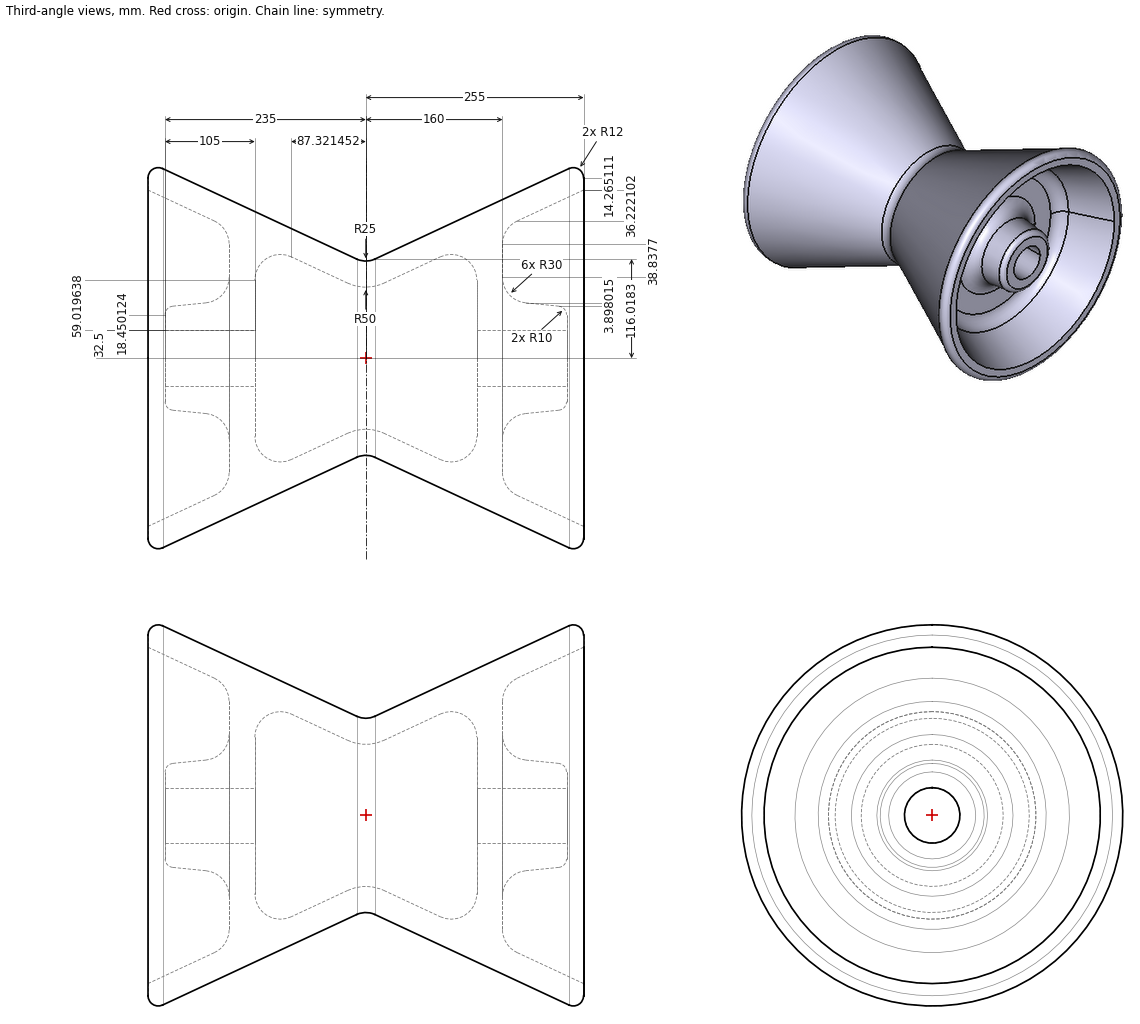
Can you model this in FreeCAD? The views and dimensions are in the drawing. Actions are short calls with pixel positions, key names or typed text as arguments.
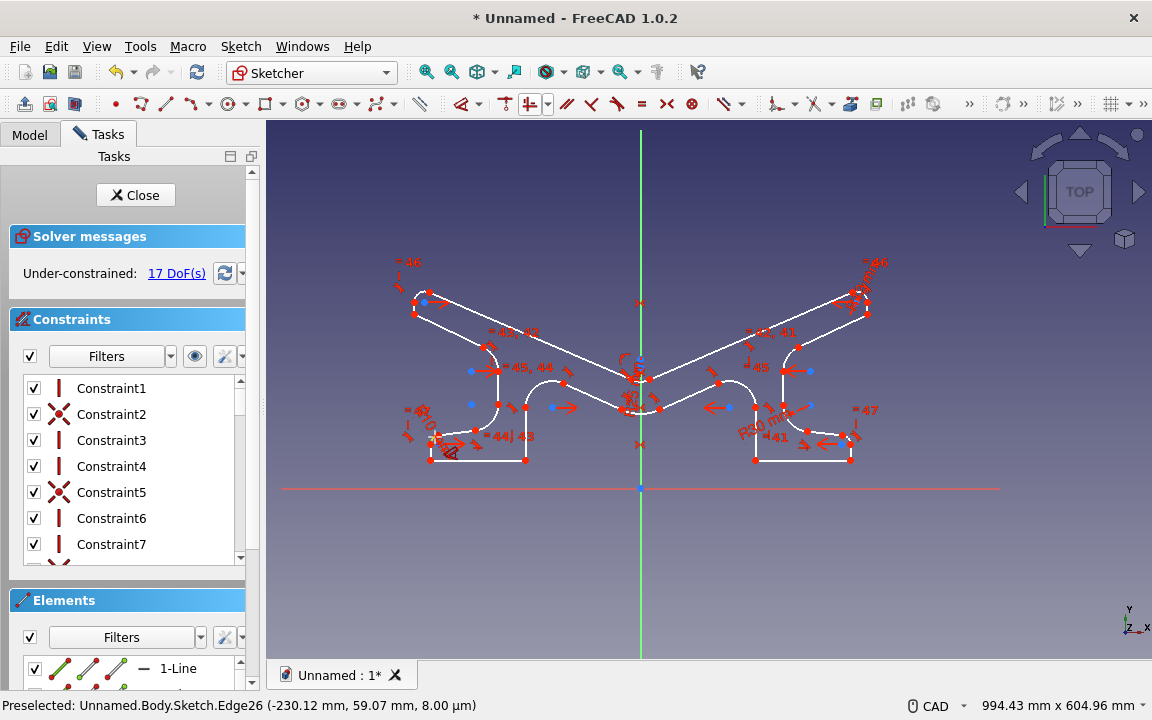
scroll(633, 413, up, 3)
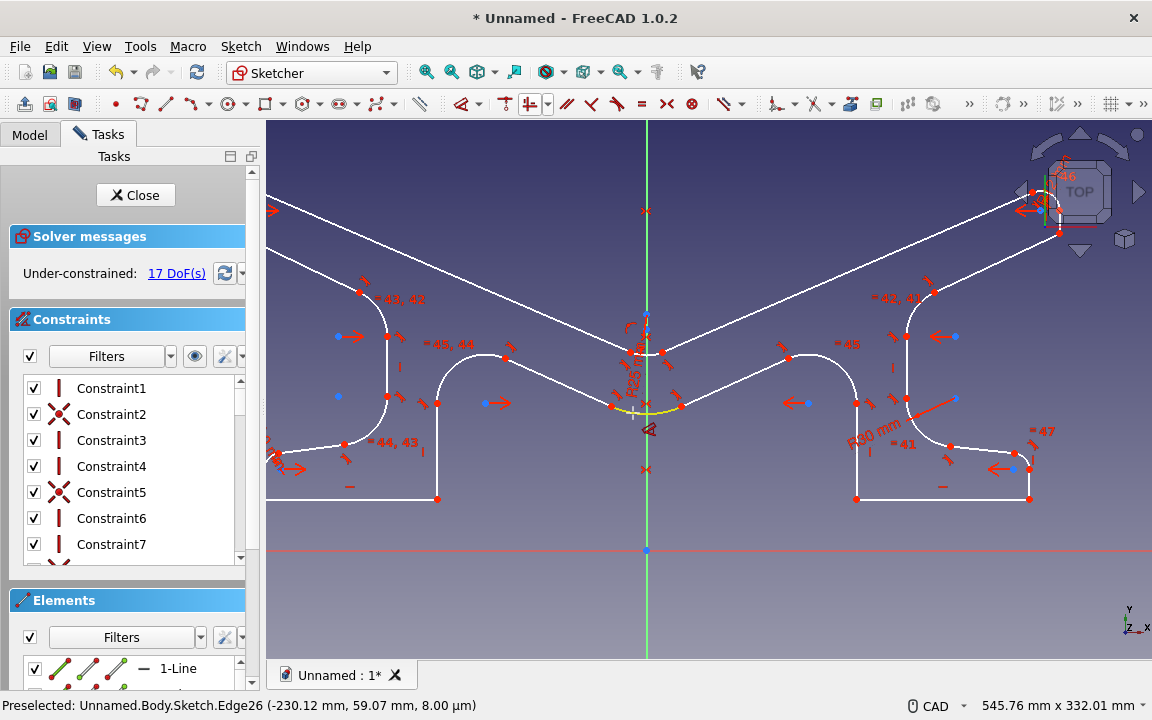
click(633, 413)
click(628, 445)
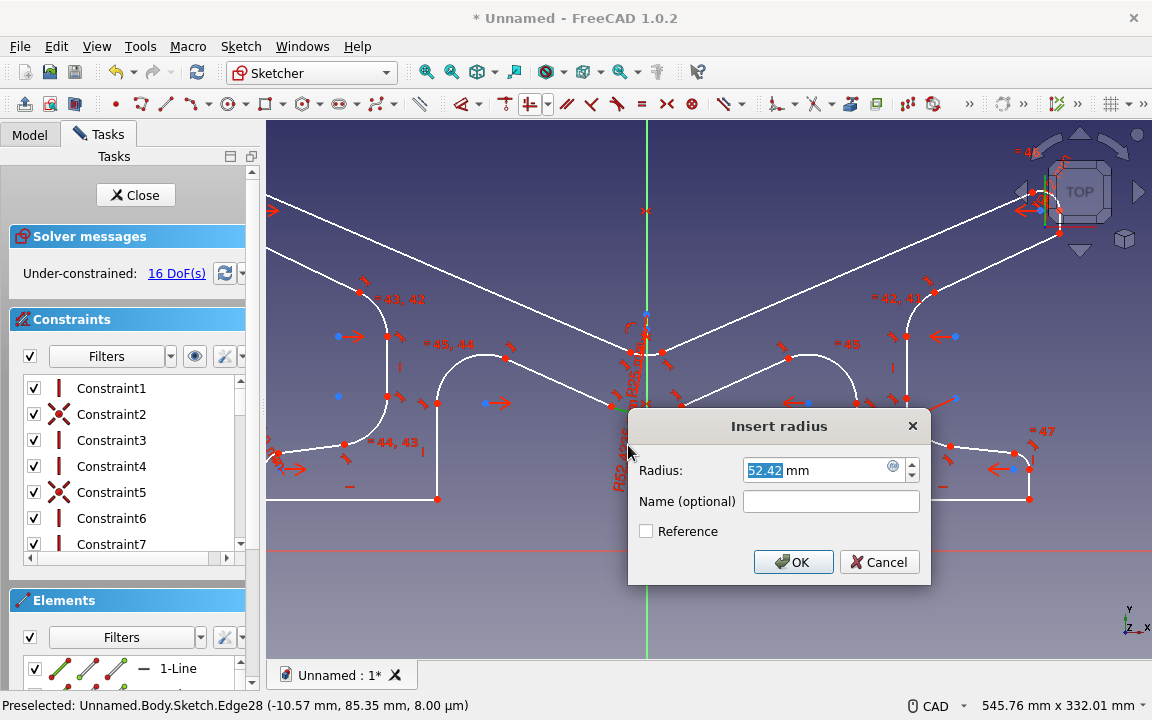
text(50)
key(Return)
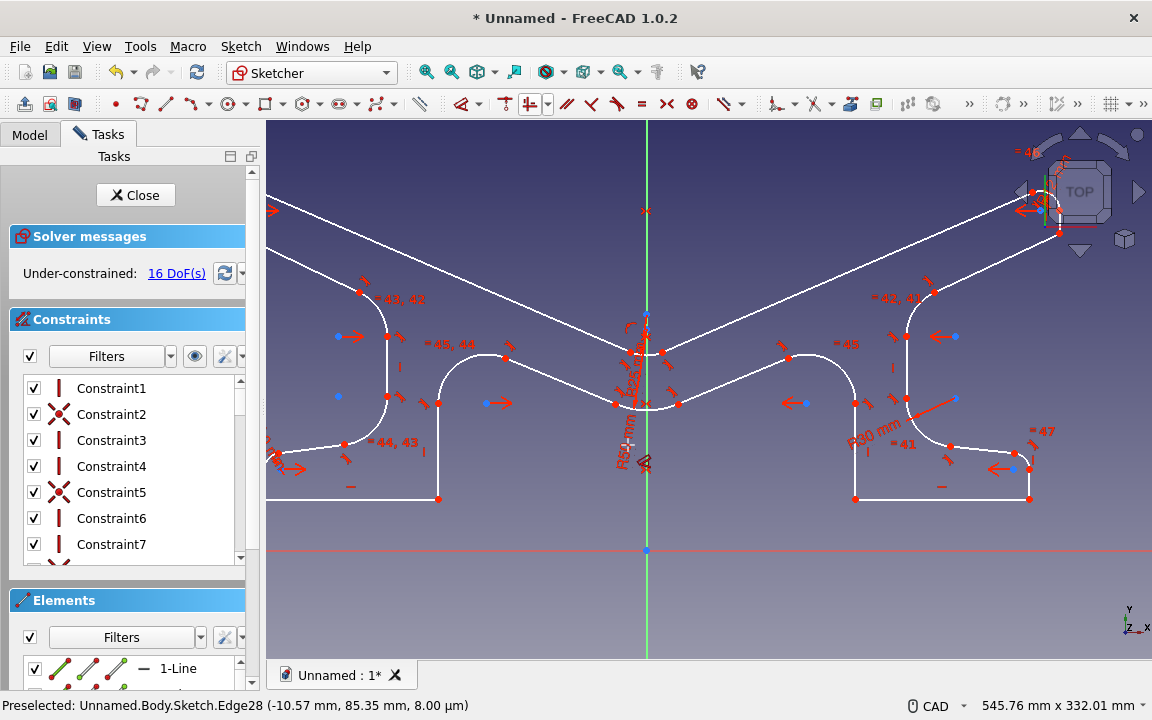
click(317, 500)
click(366, 534)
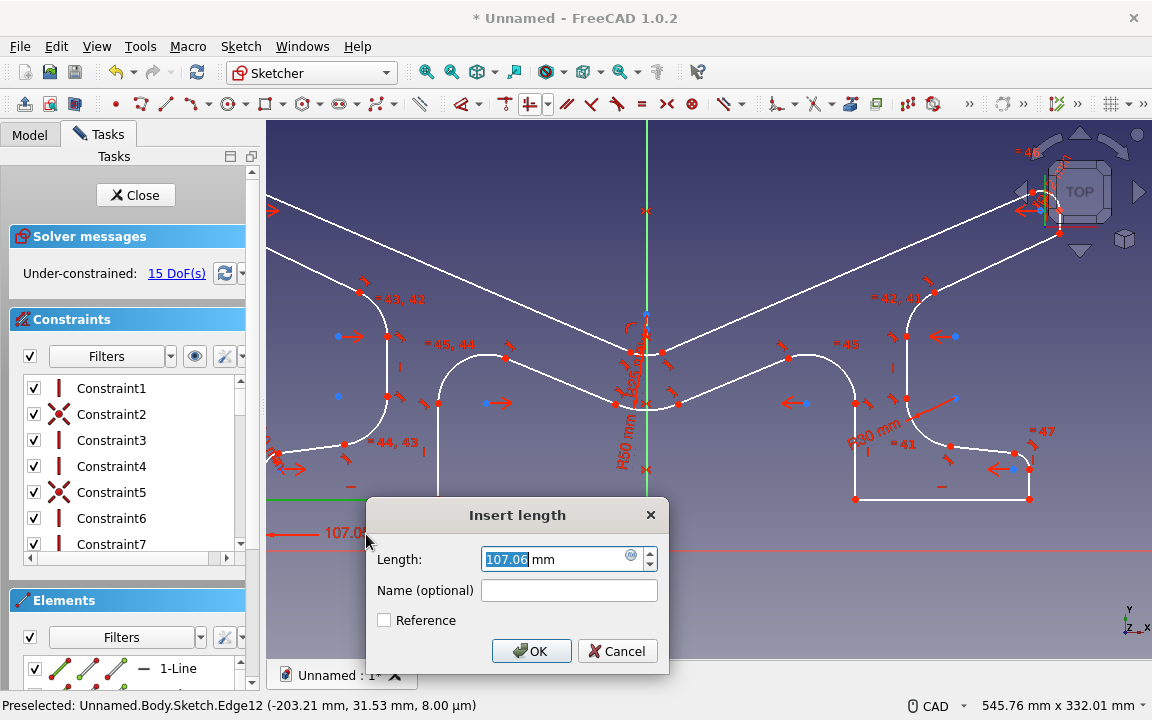
text(105)
key(Return)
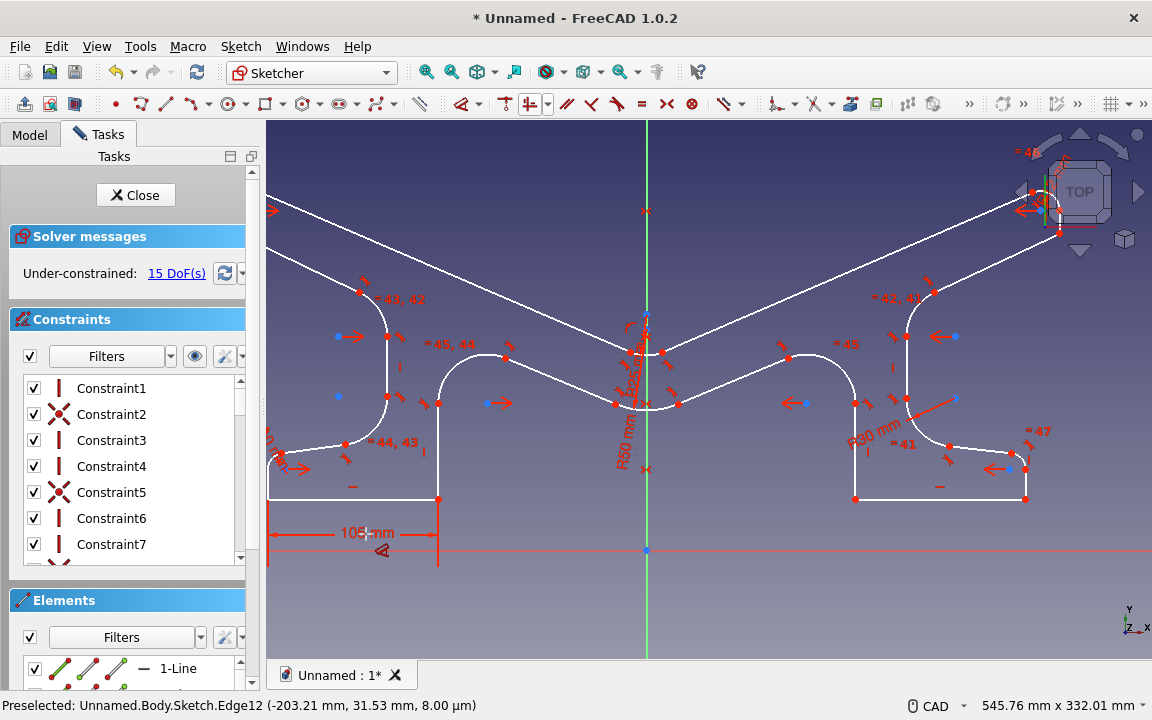
click(907, 398)
click(777, 585)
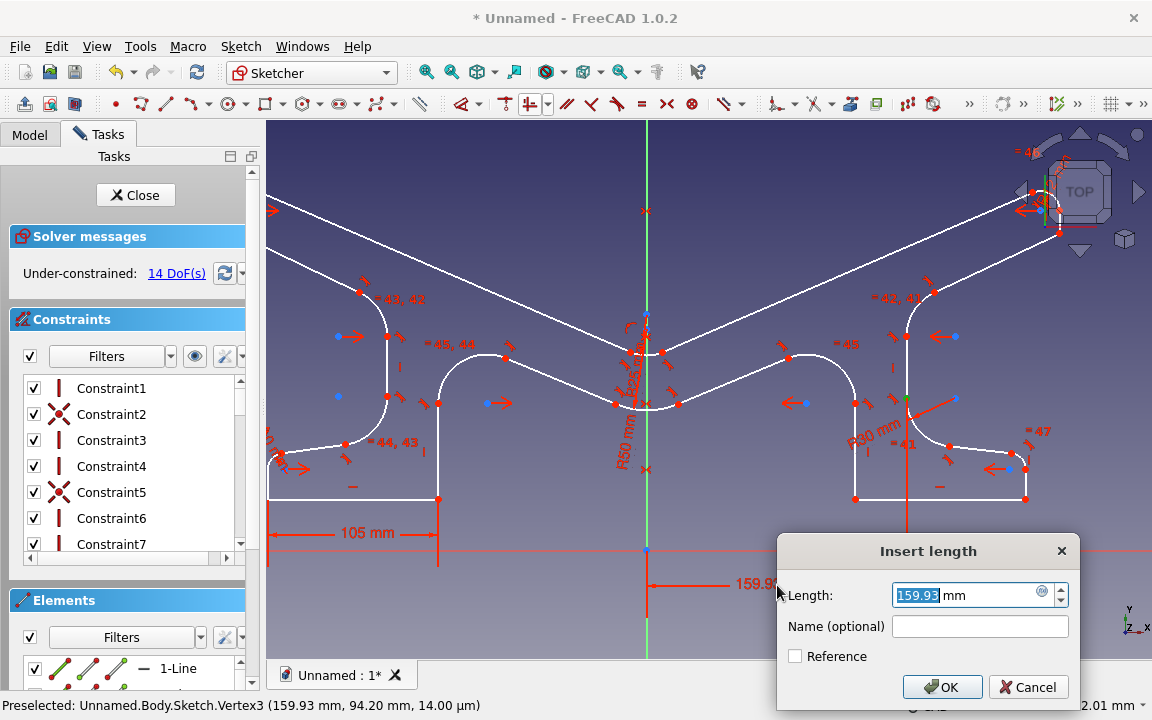
text(160)
key(Return)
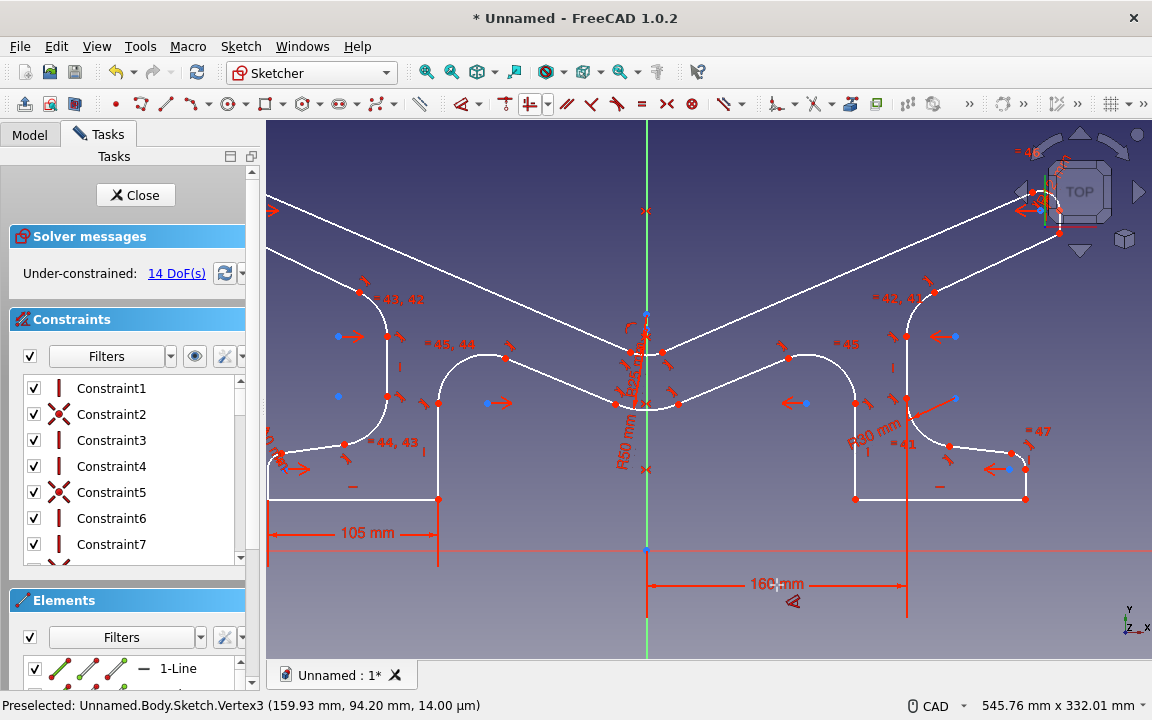
scroll(633, 412, down, 3)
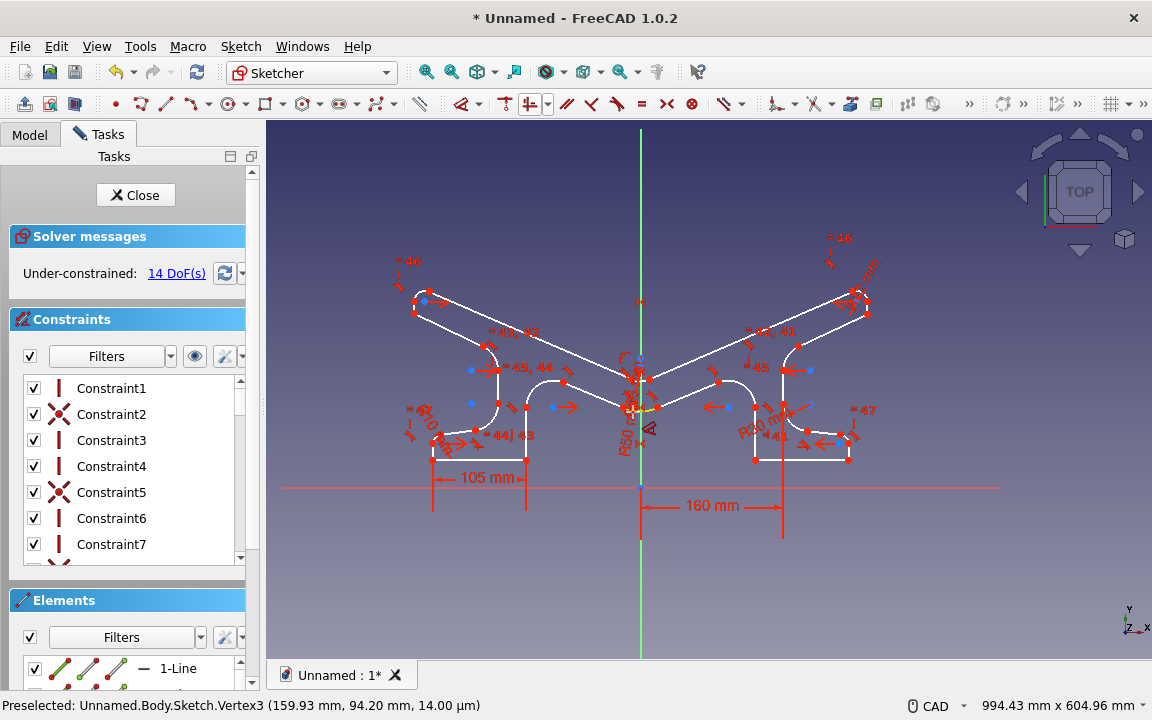
click(867, 314)
click(806, 522)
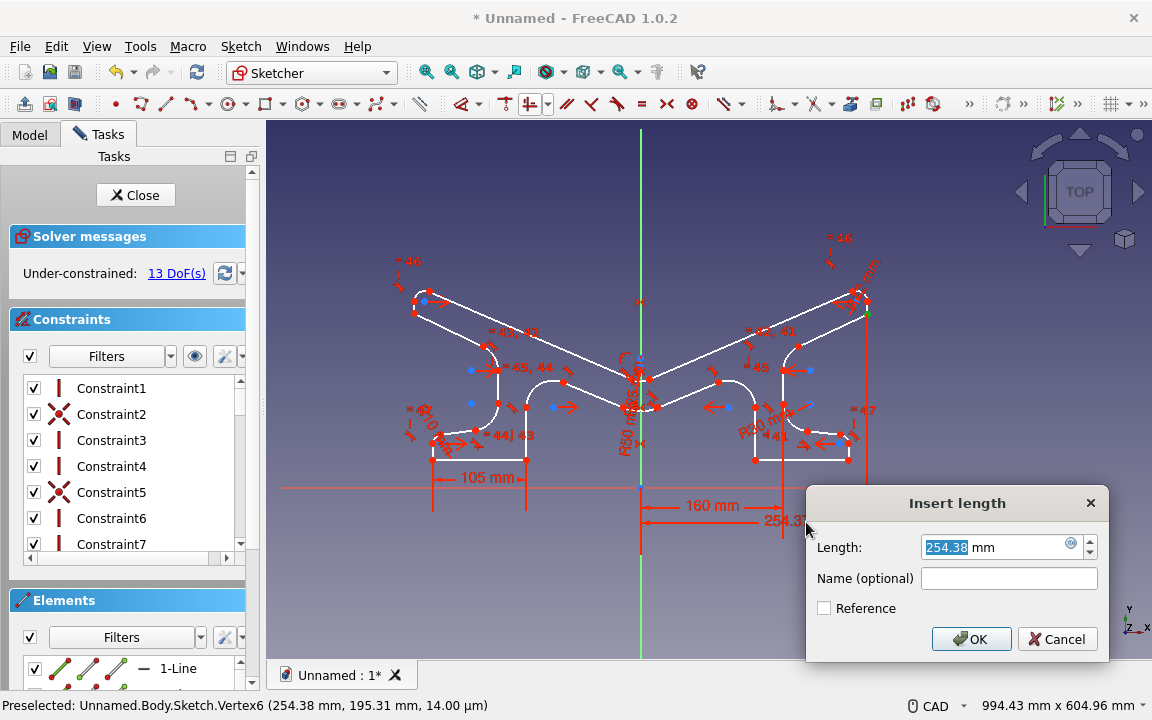
text(255)
key(Return)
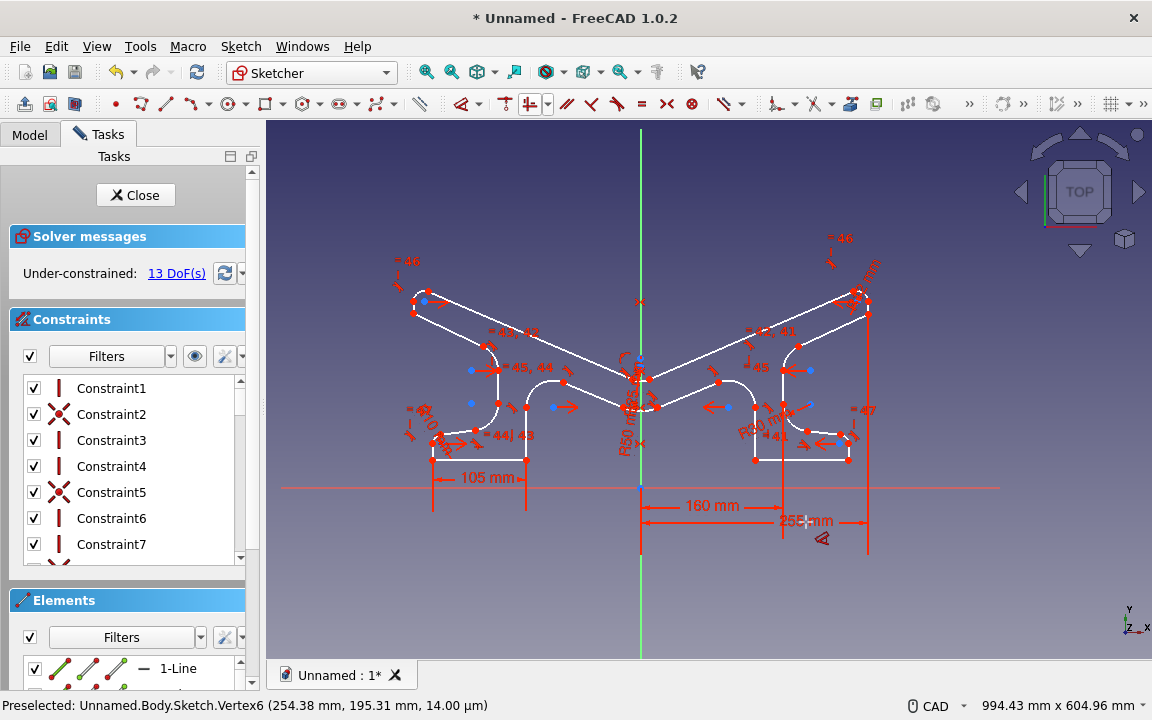
scroll(433, 444, up, 2)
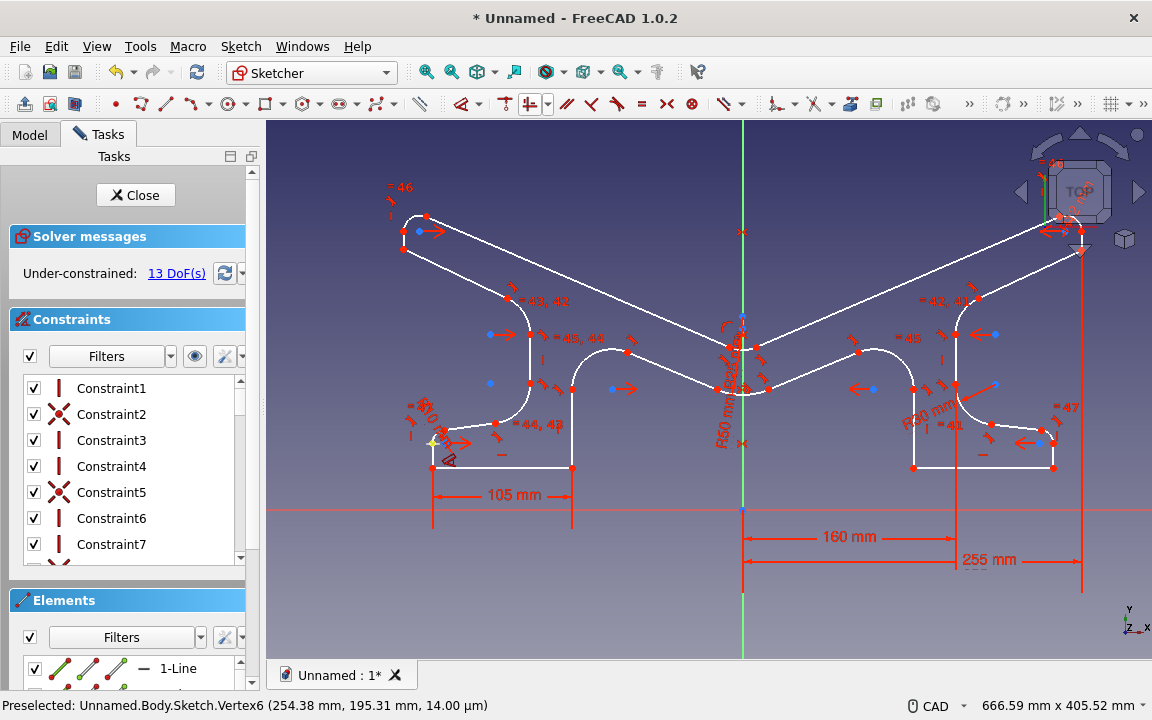
click(433, 443)
click(588, 544)